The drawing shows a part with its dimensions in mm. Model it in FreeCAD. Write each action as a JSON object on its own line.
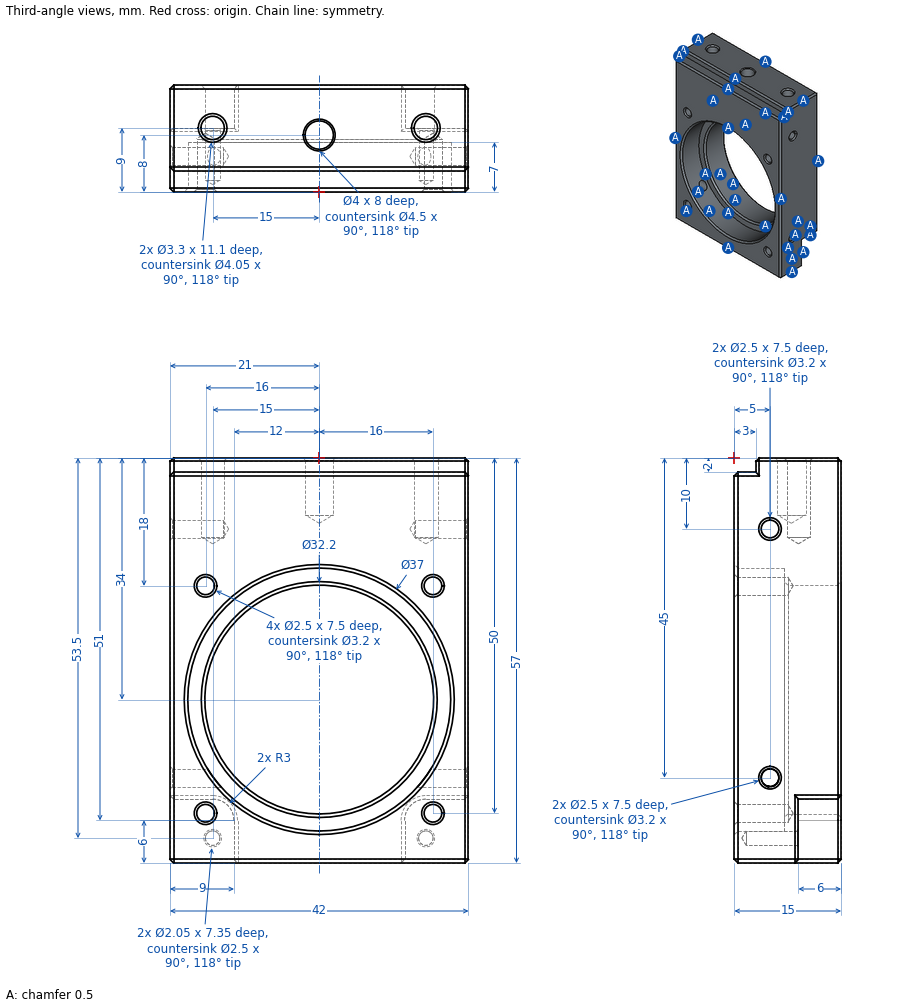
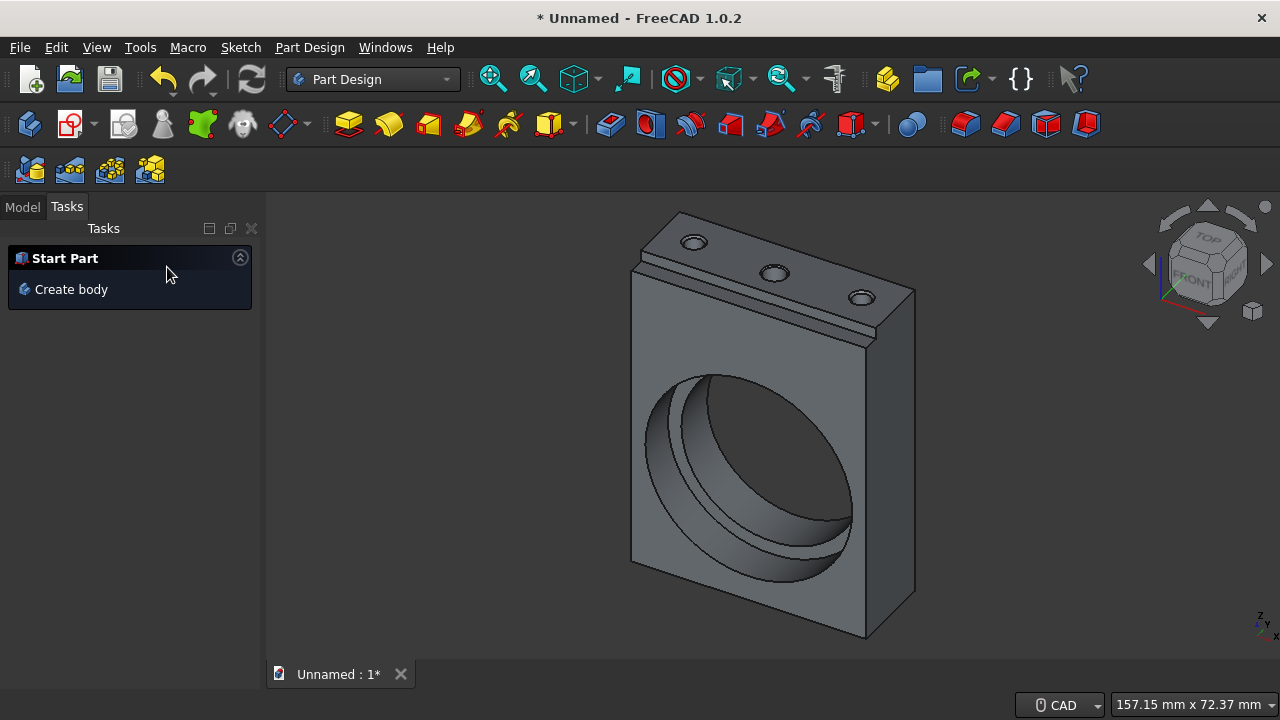
{"action": "left_click", "coordinate": [70, 124]}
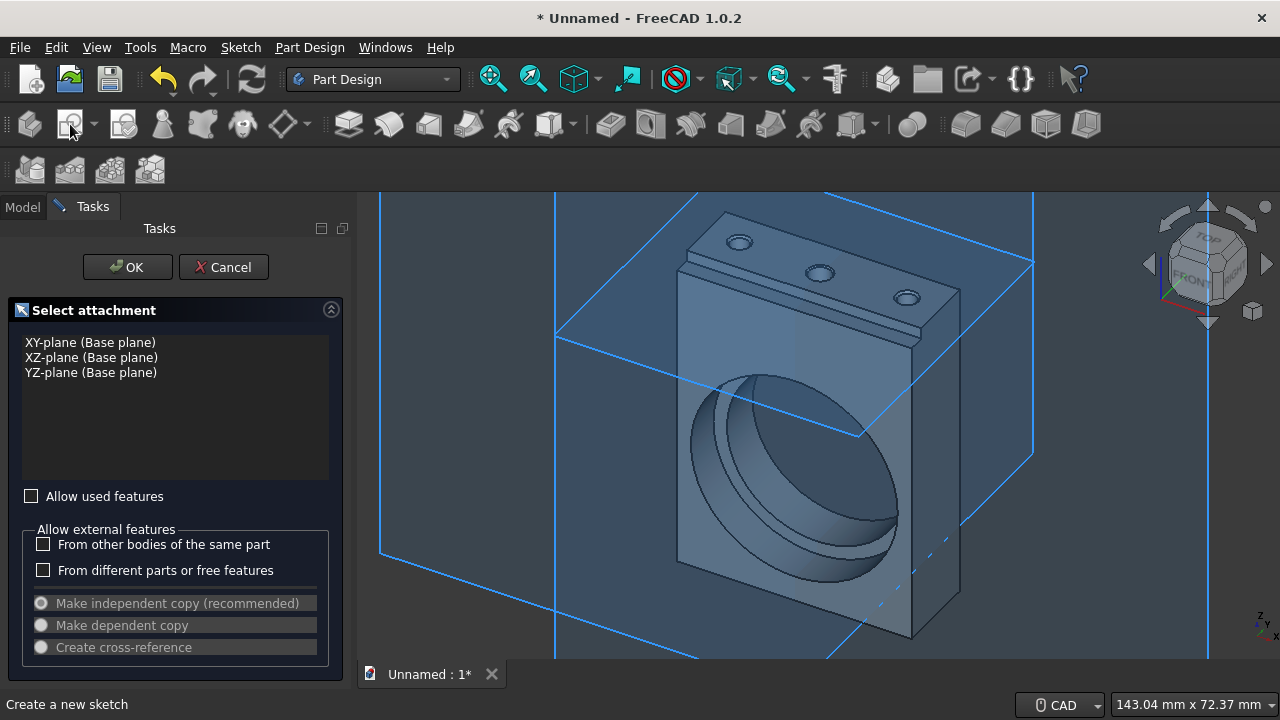
{"action": "left_click", "coordinate": [82, 358]}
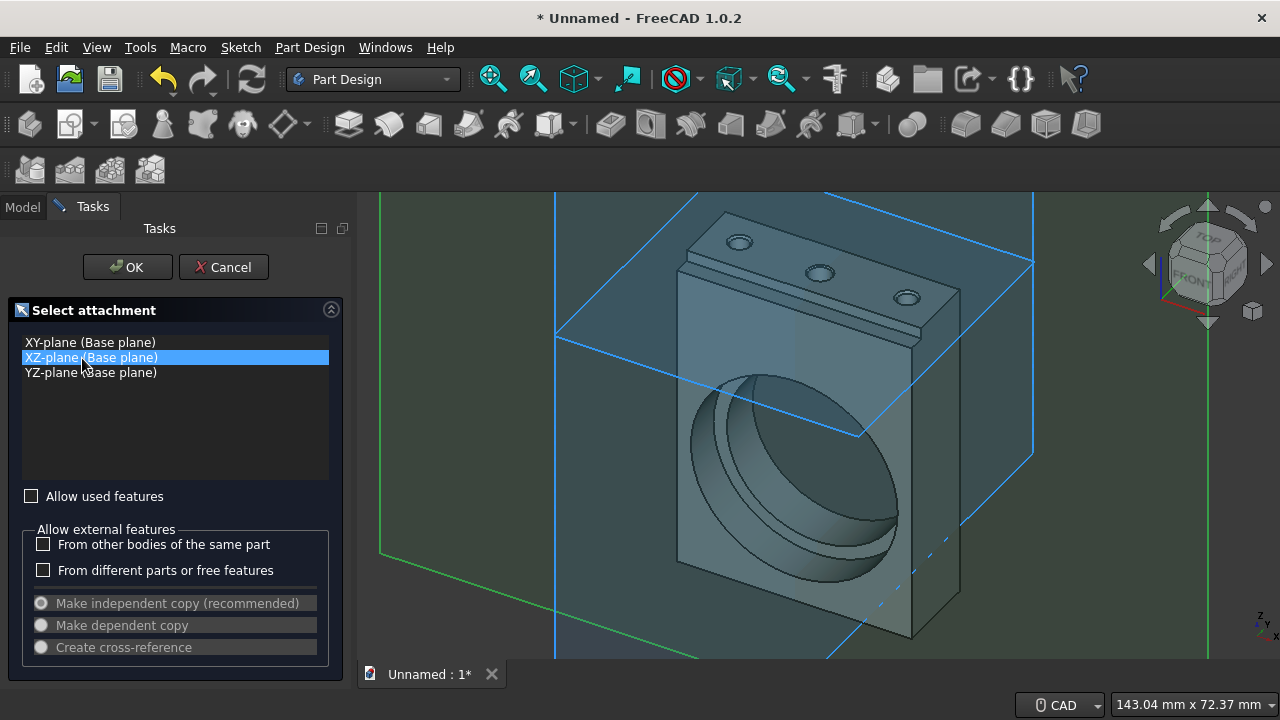
{"action": "left_click", "coordinate": [128, 267]}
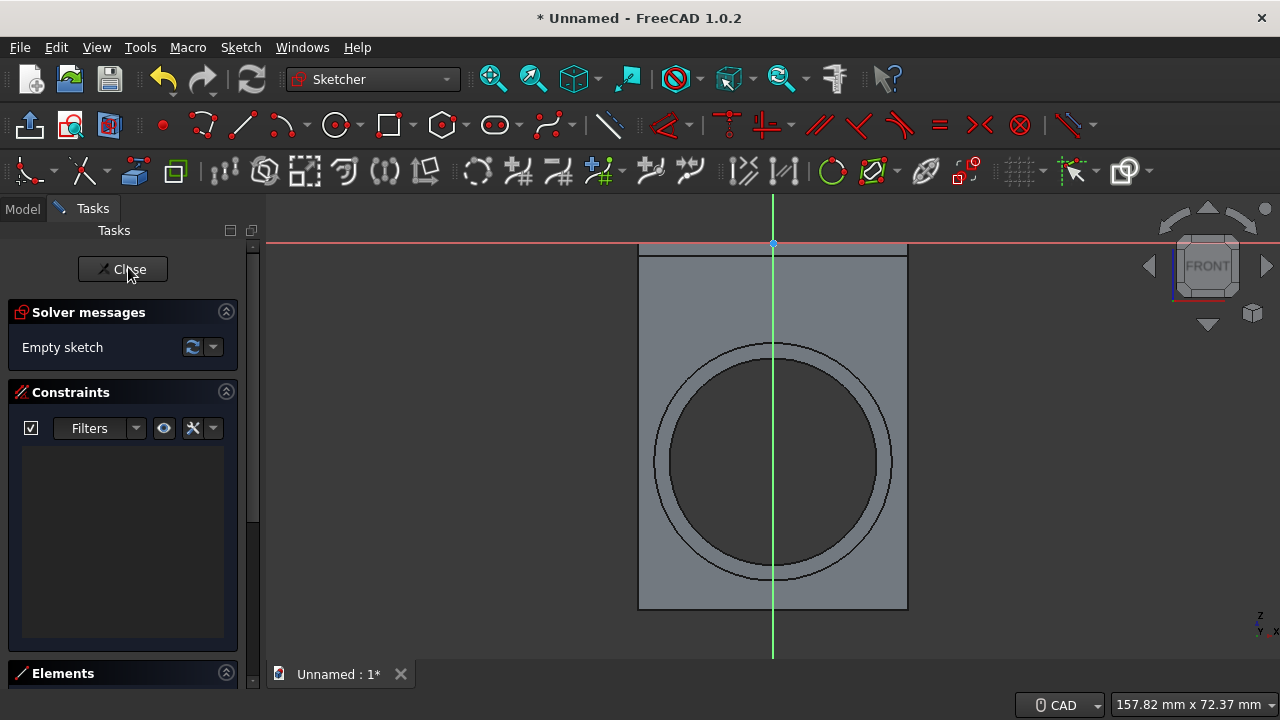
{"action": "scroll", "coordinate": [395, 510], "scroll_direction": "down", "scroll_amount": 1}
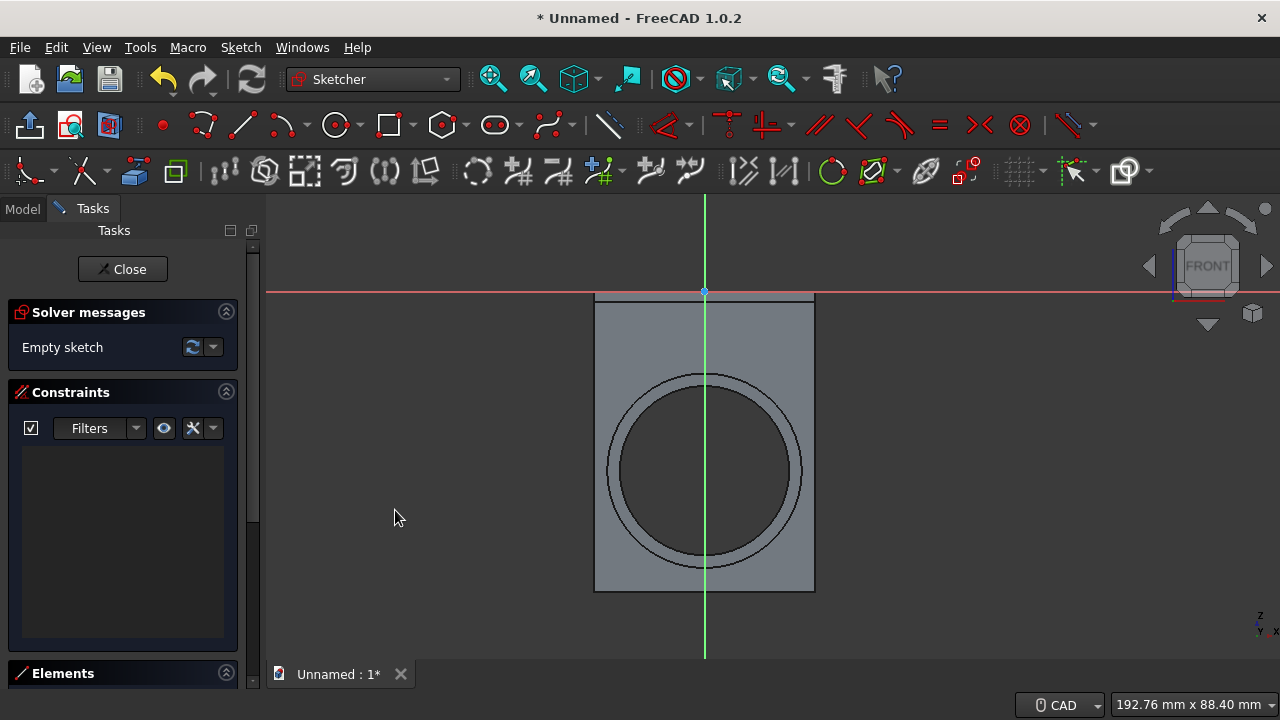
{"action": "key", "text": "g c"}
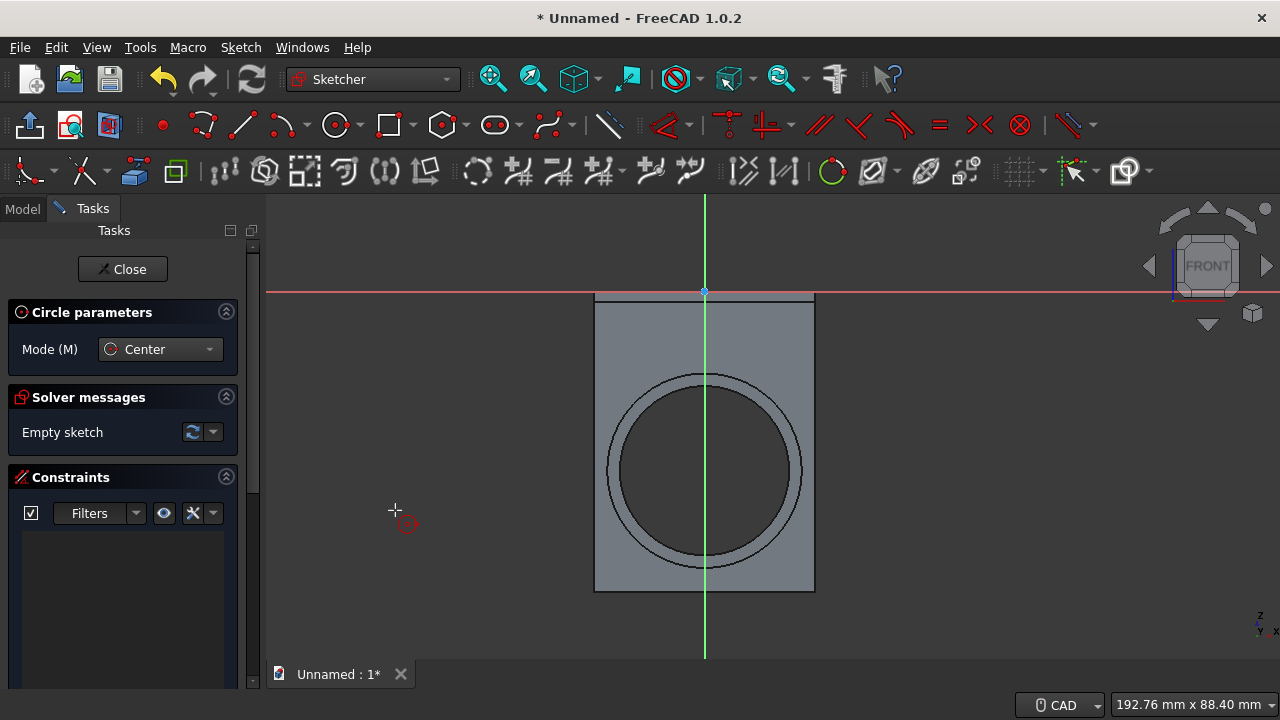
{"action": "scroll", "coordinate": [620, 387], "scroll_direction": "up", "scroll_amount": 7}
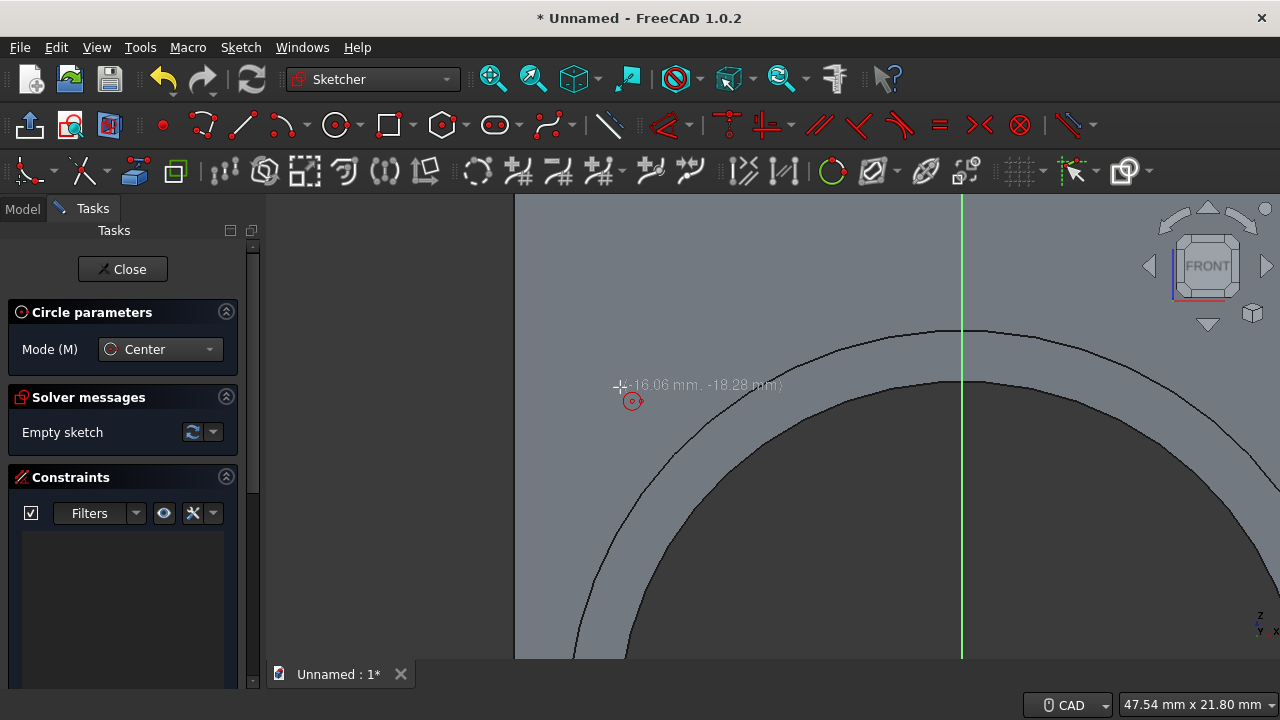
{"action": "scroll", "coordinate": [620, 387], "scroll_direction": "down", "scroll_amount": 7}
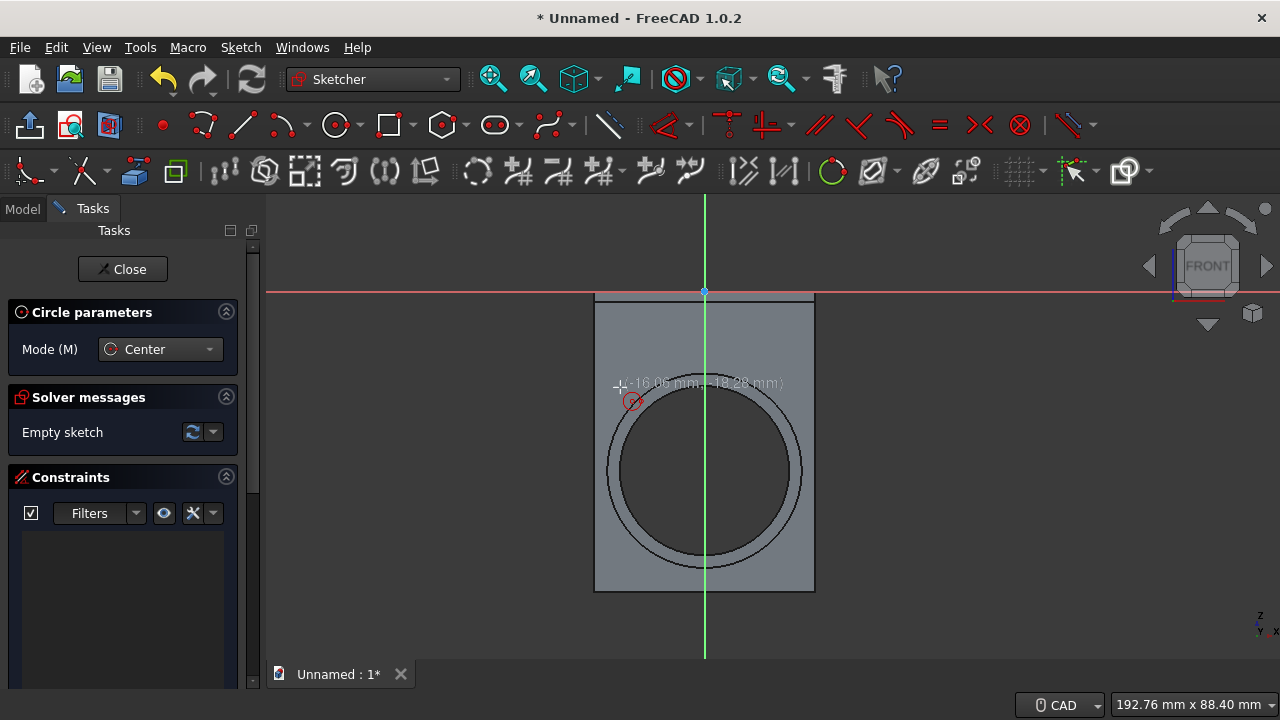
{"action": "left_click", "coordinate": [620, 387]}
{"action": "mouse_move", "coordinate": [625, 382]}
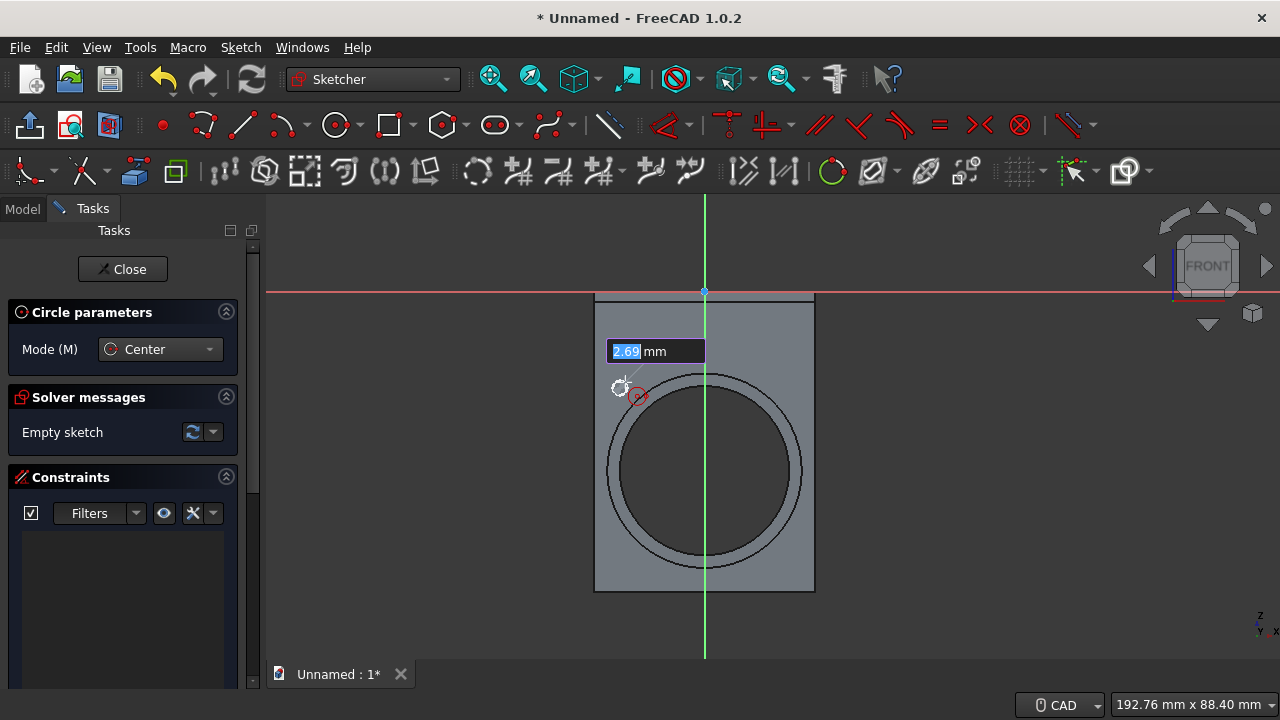
{"action": "type", "text": "2.5"}
{"action": "key", "text": "Return"}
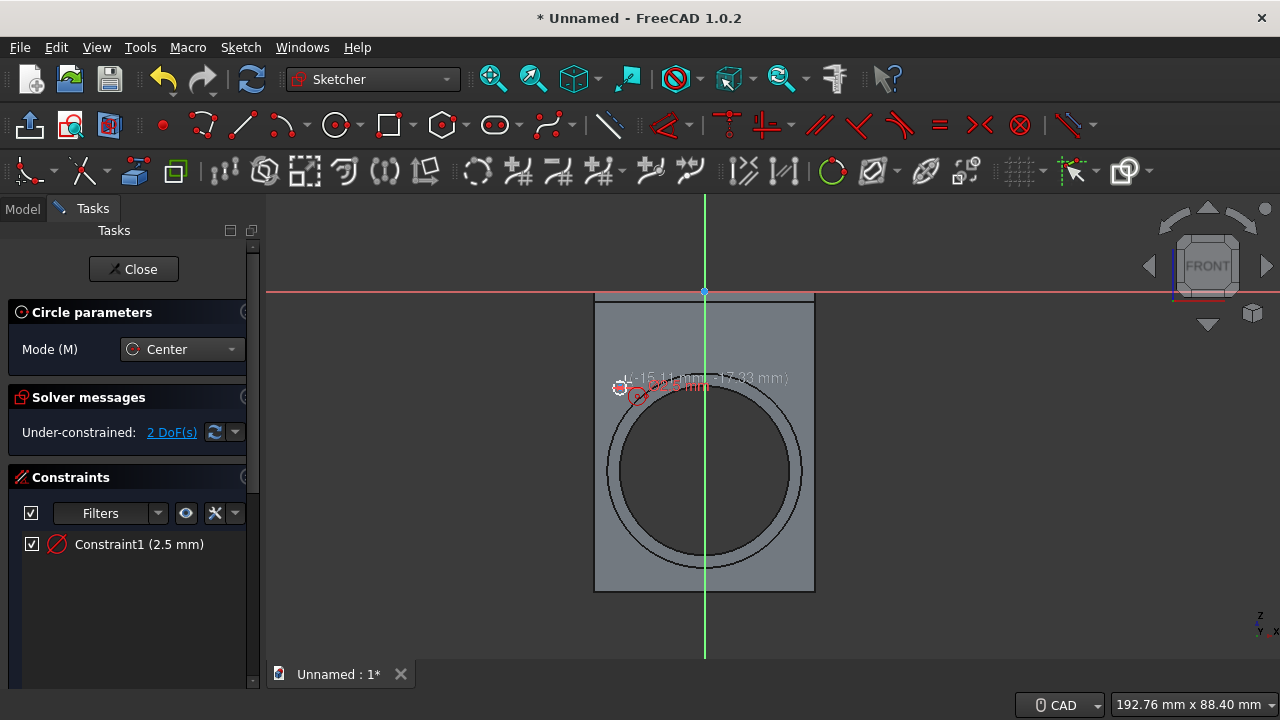
{"action": "scroll", "coordinate": [789, 387], "scroll_direction": "up", "scroll_amount": 7}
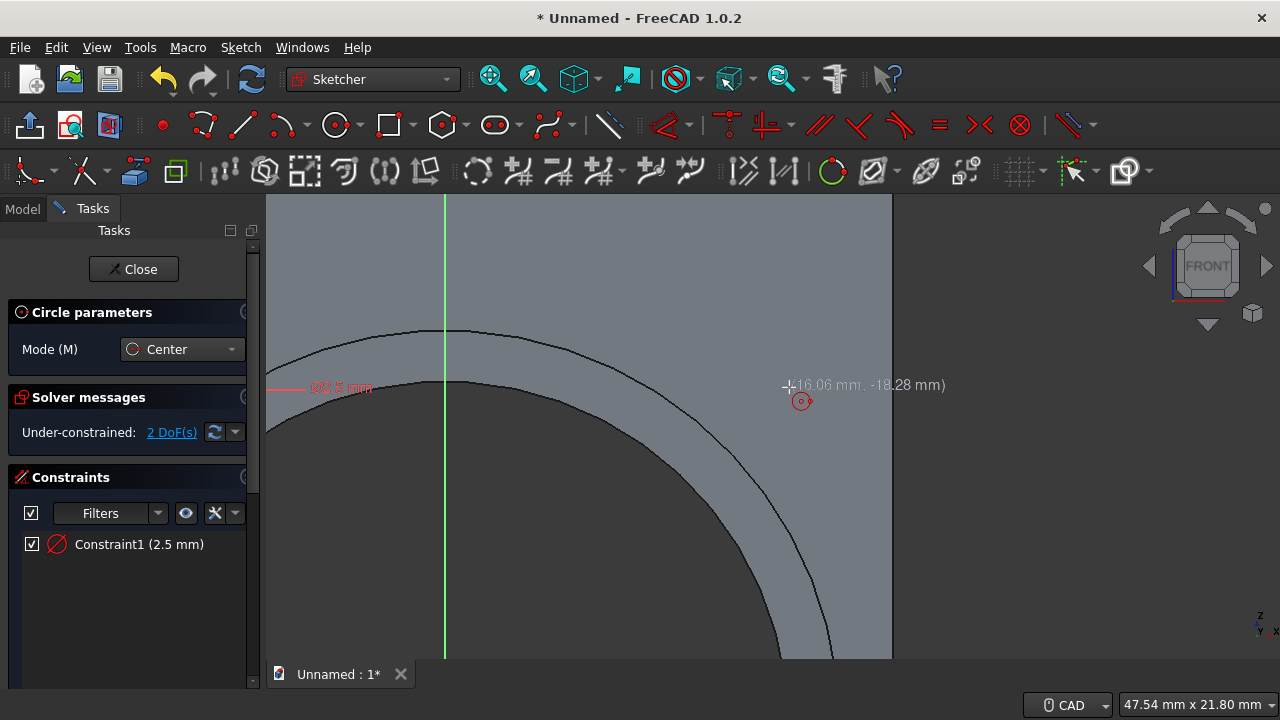
{"action": "scroll", "coordinate": [790, 387], "scroll_direction": "down", "scroll_amount": 7}